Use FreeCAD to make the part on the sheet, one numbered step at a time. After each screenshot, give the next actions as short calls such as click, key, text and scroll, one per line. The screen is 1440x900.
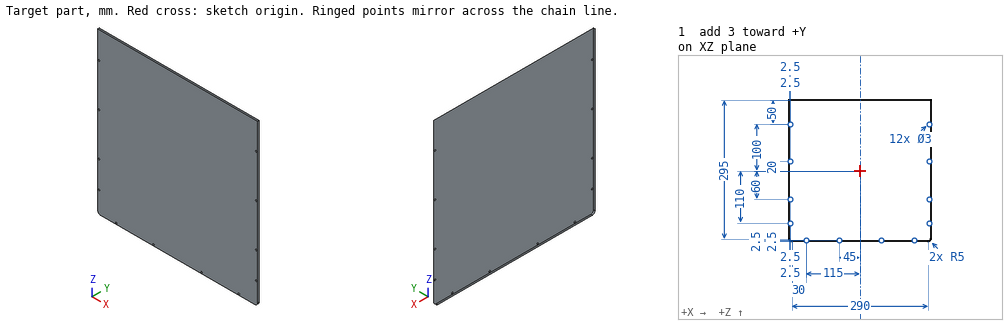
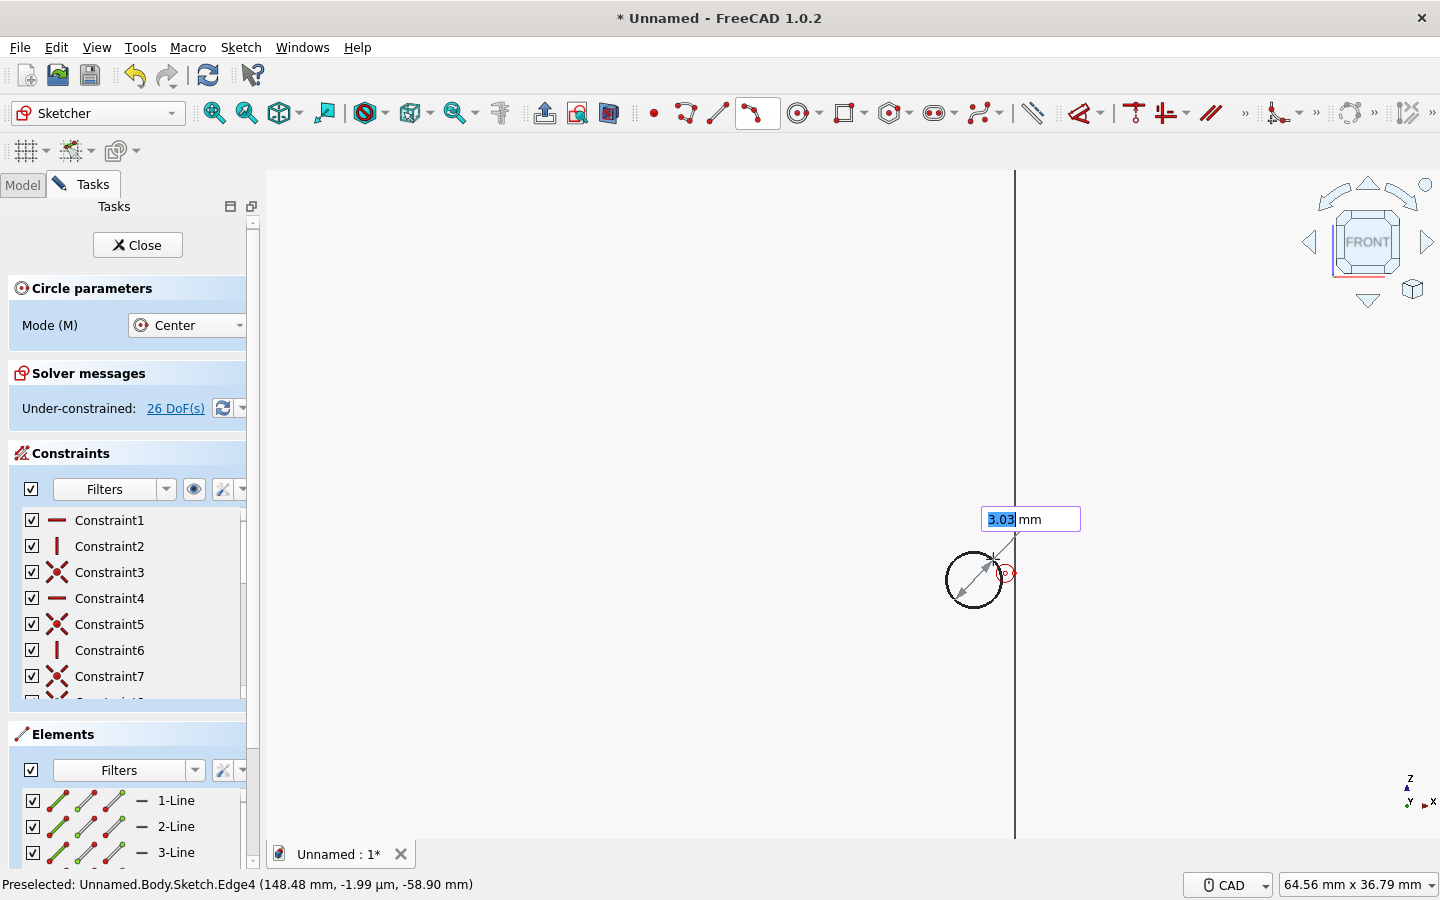
text(3)
key(Return)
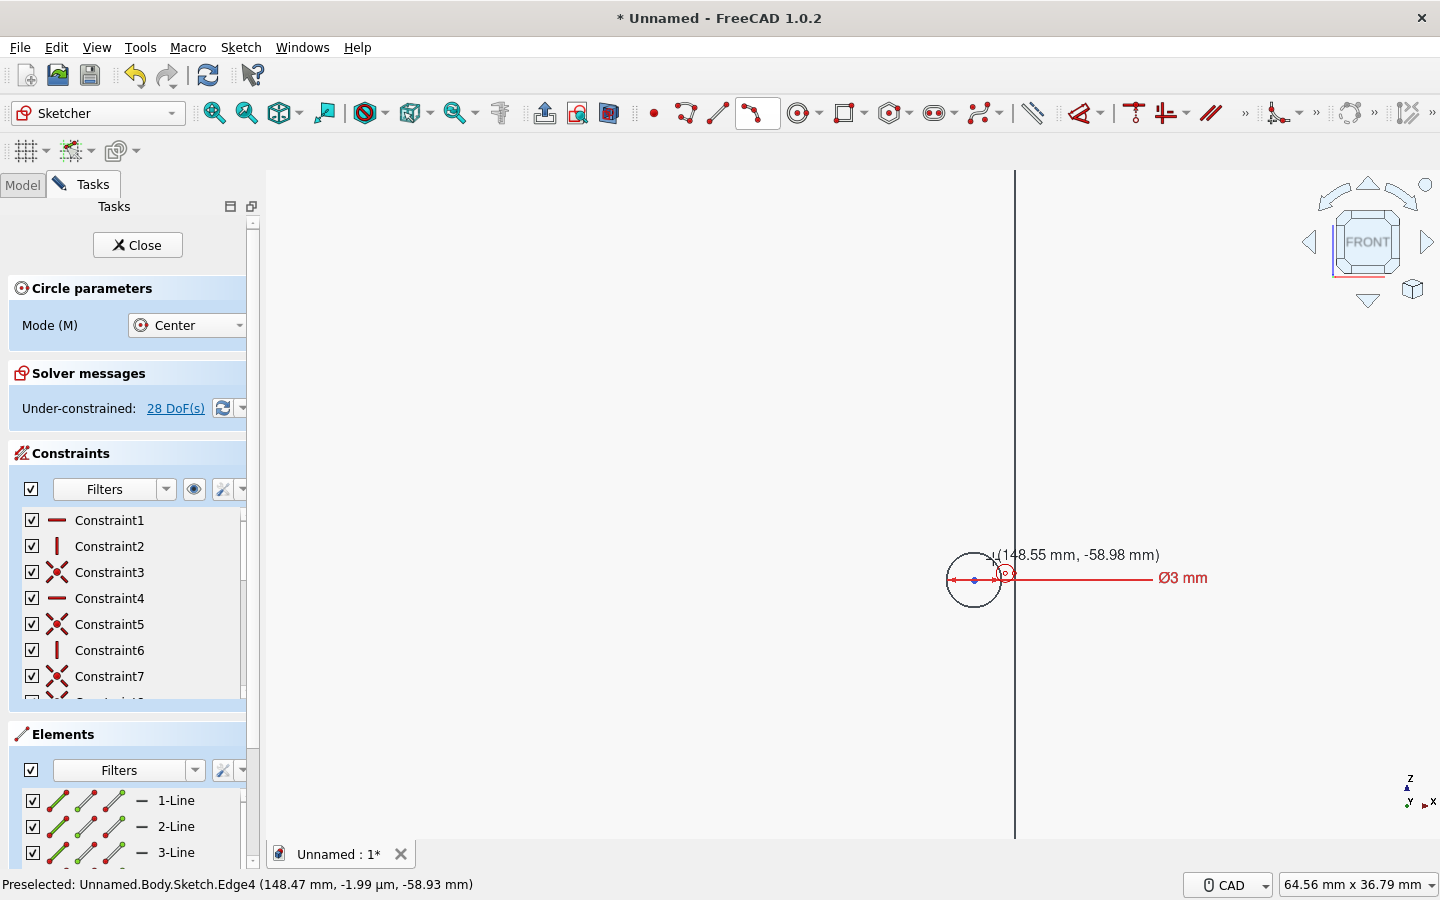
scroll(985, 586, down, 13)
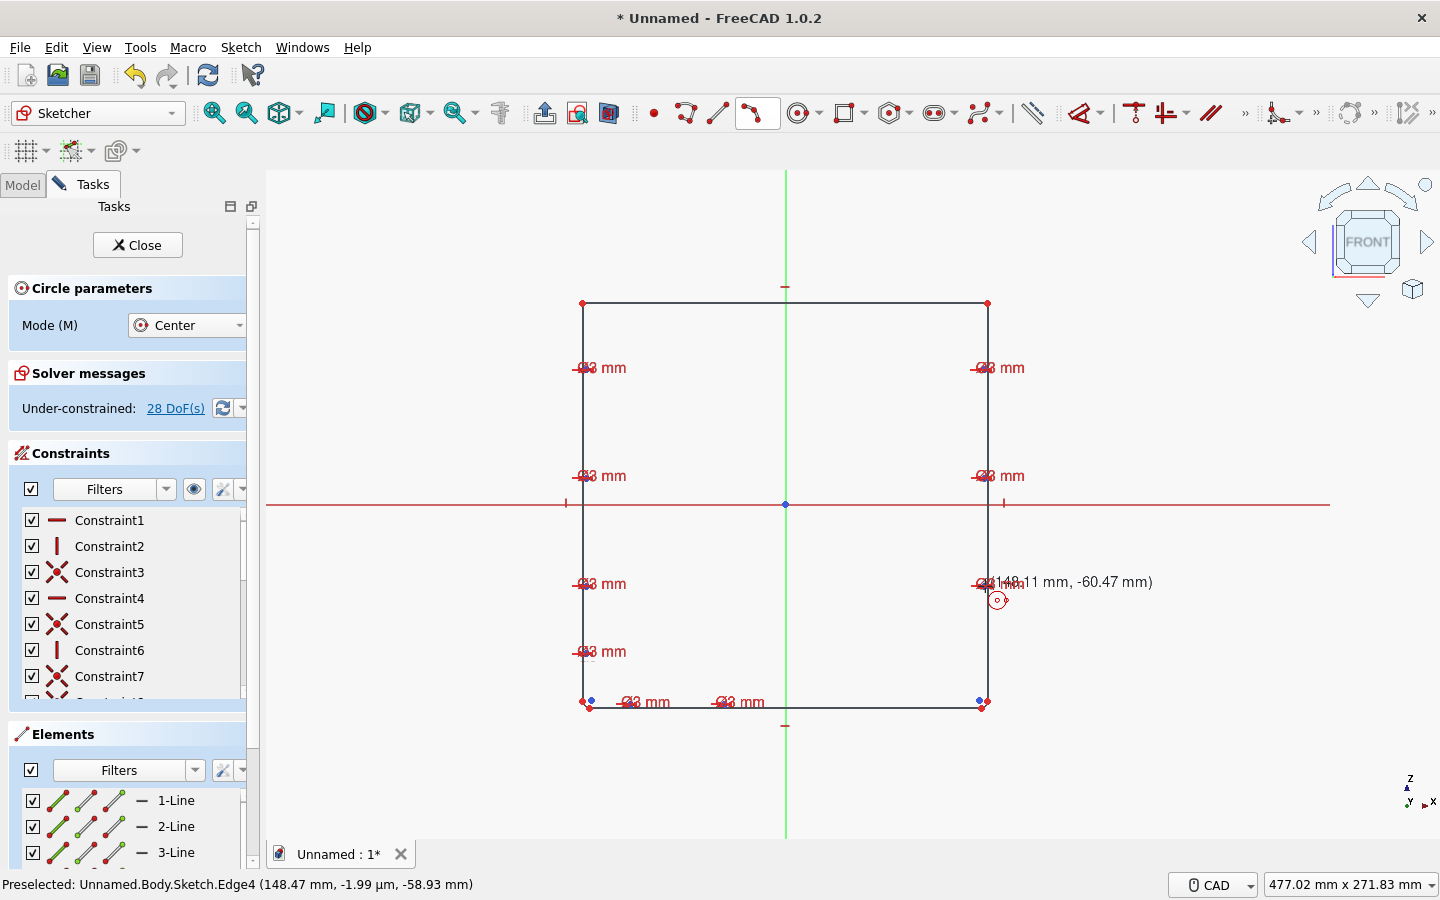
scroll(846, 704, up, 13)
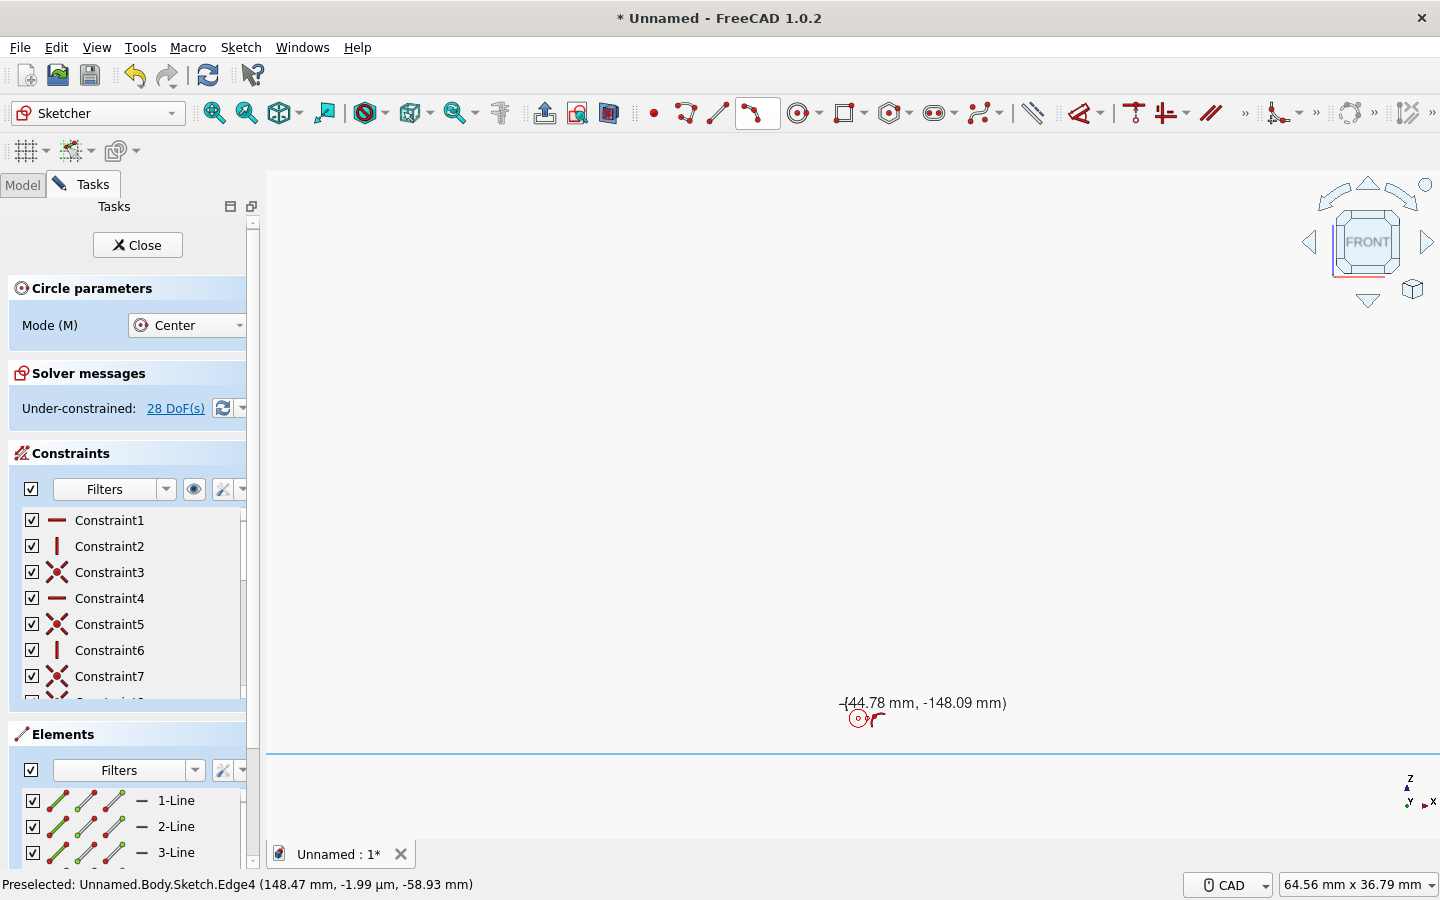
click(844, 697)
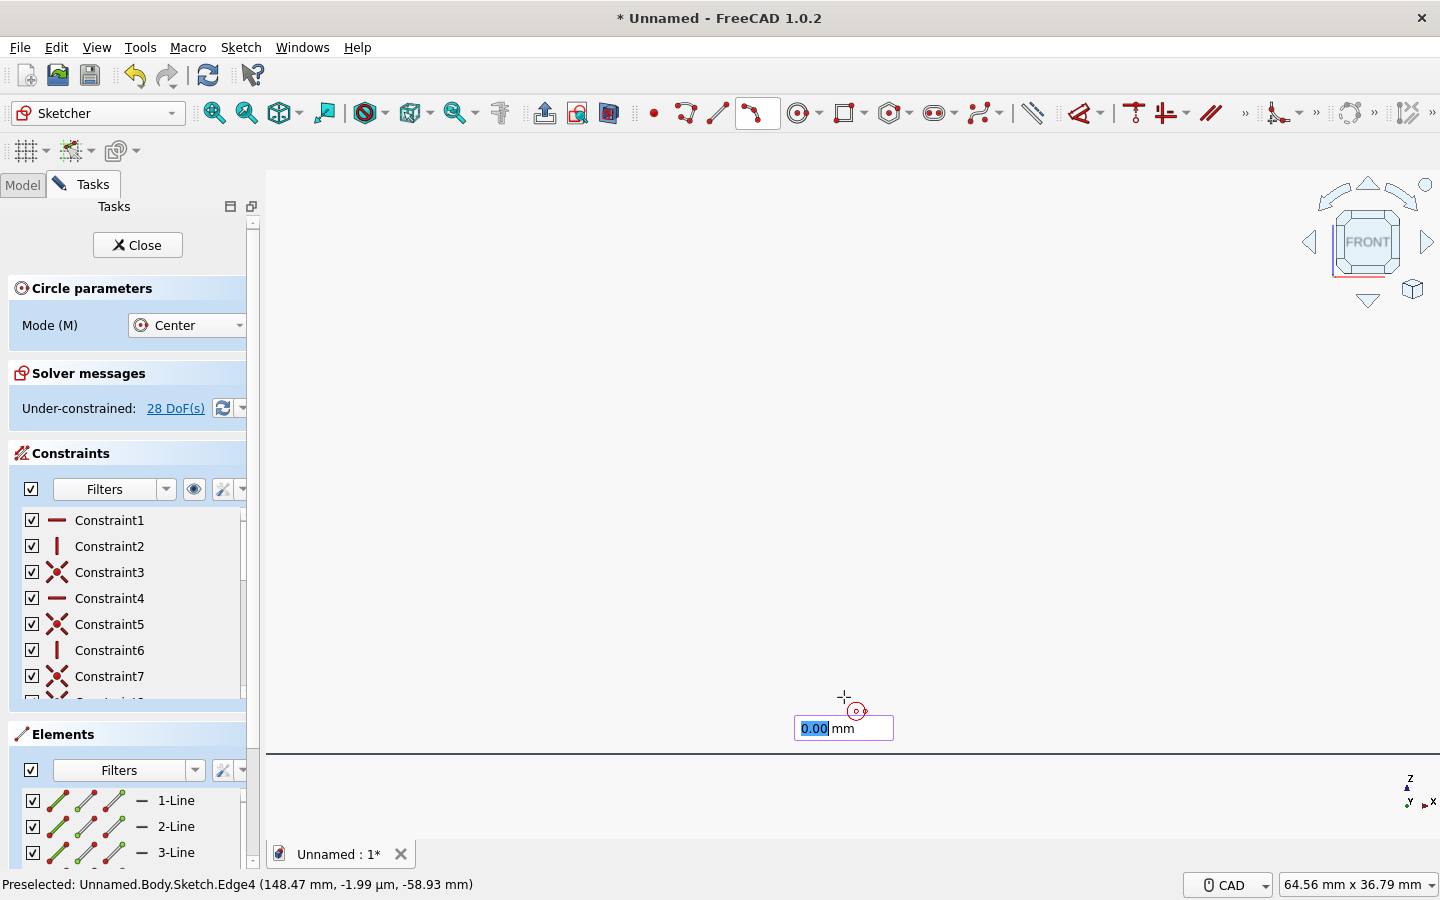
scroll(845, 704, down, 13)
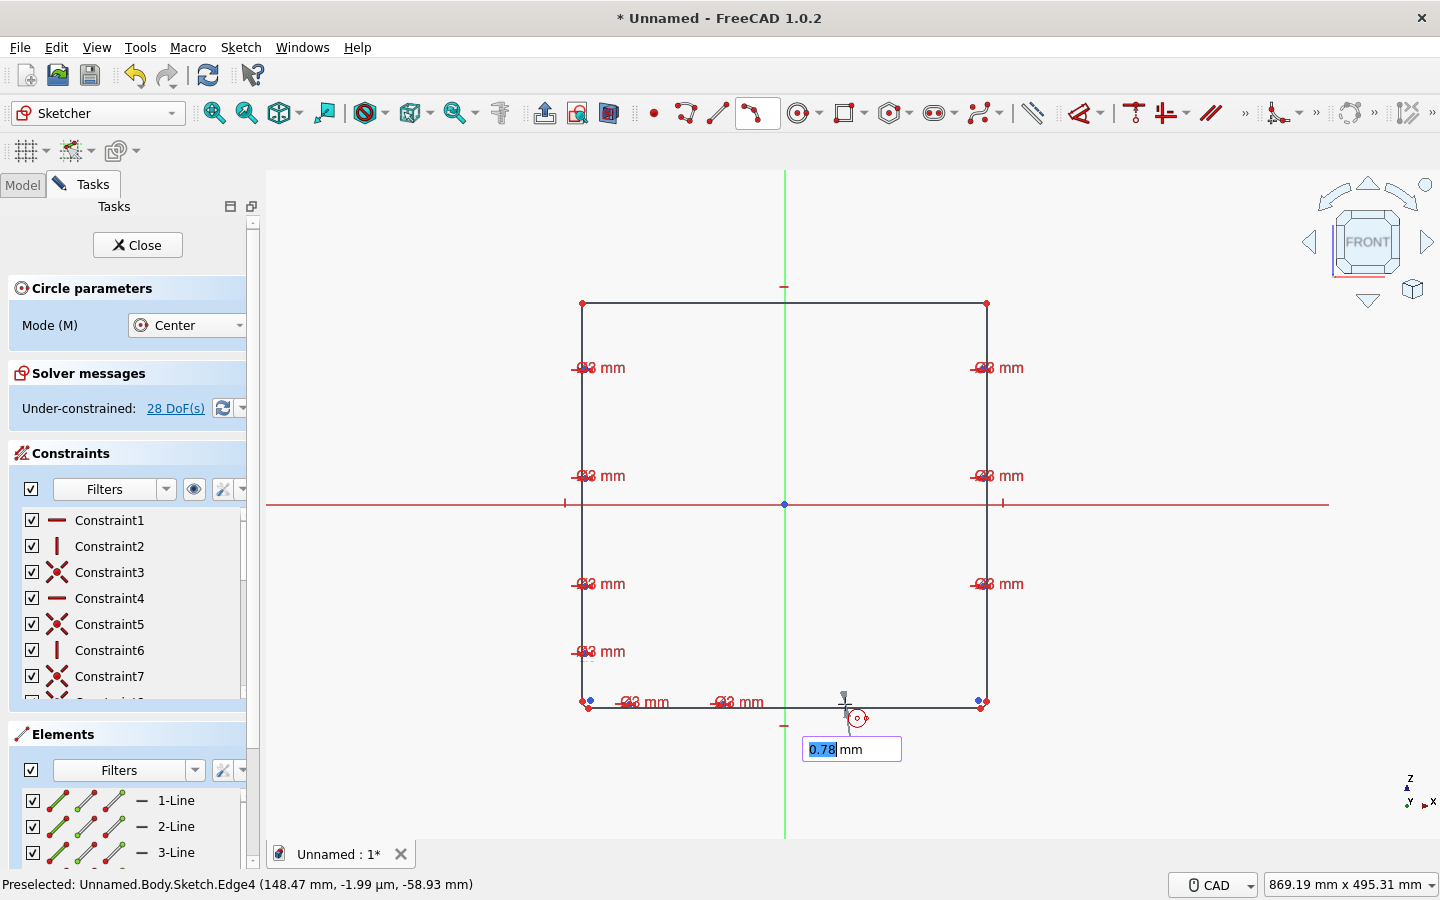
scroll(847, 703, up, 6)
move(845, 700)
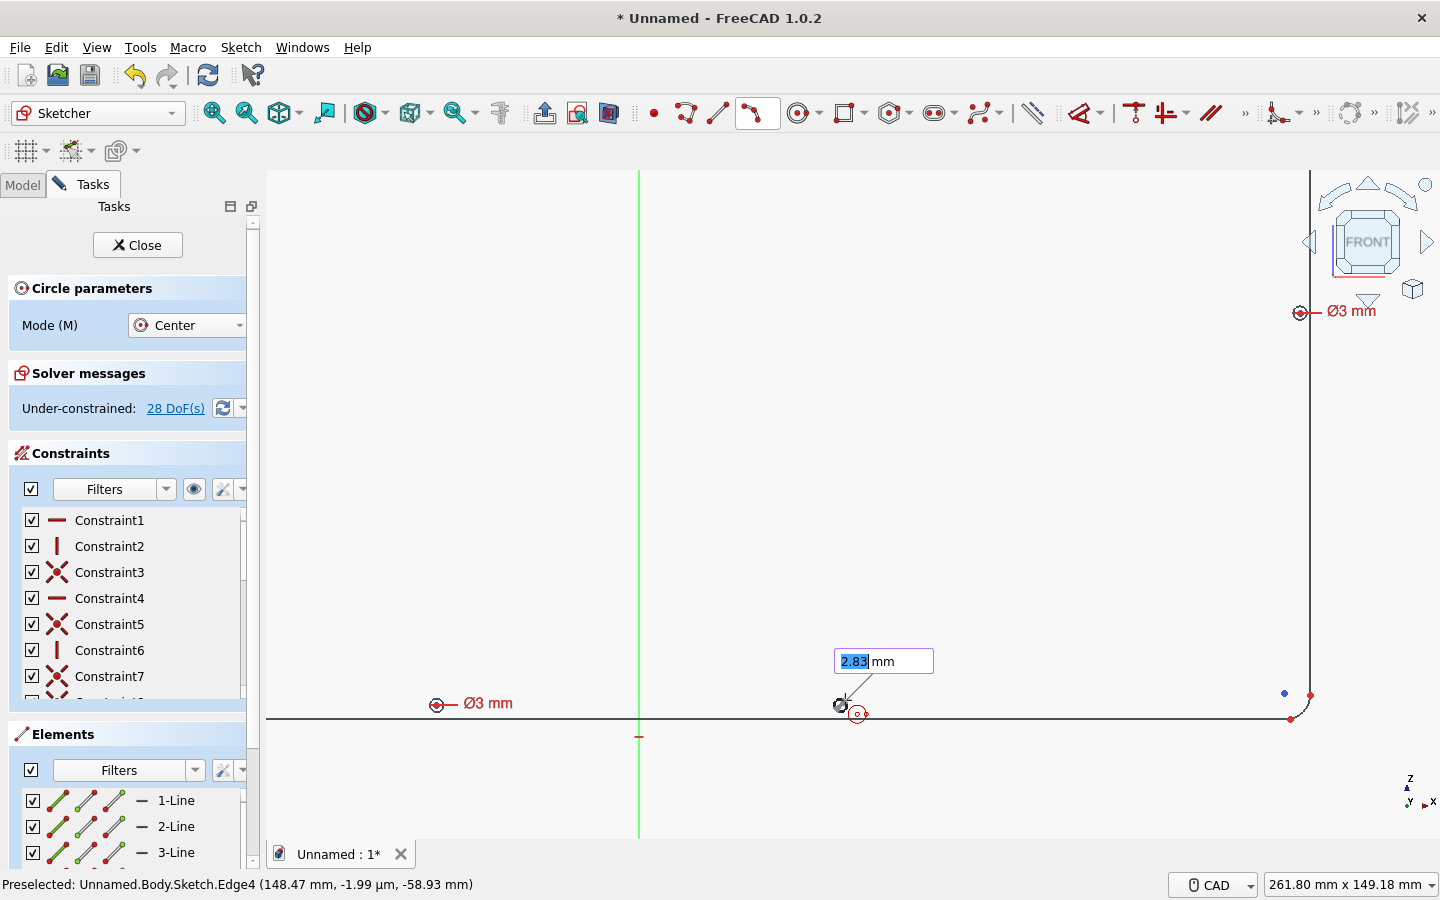
text(3)
key(Return)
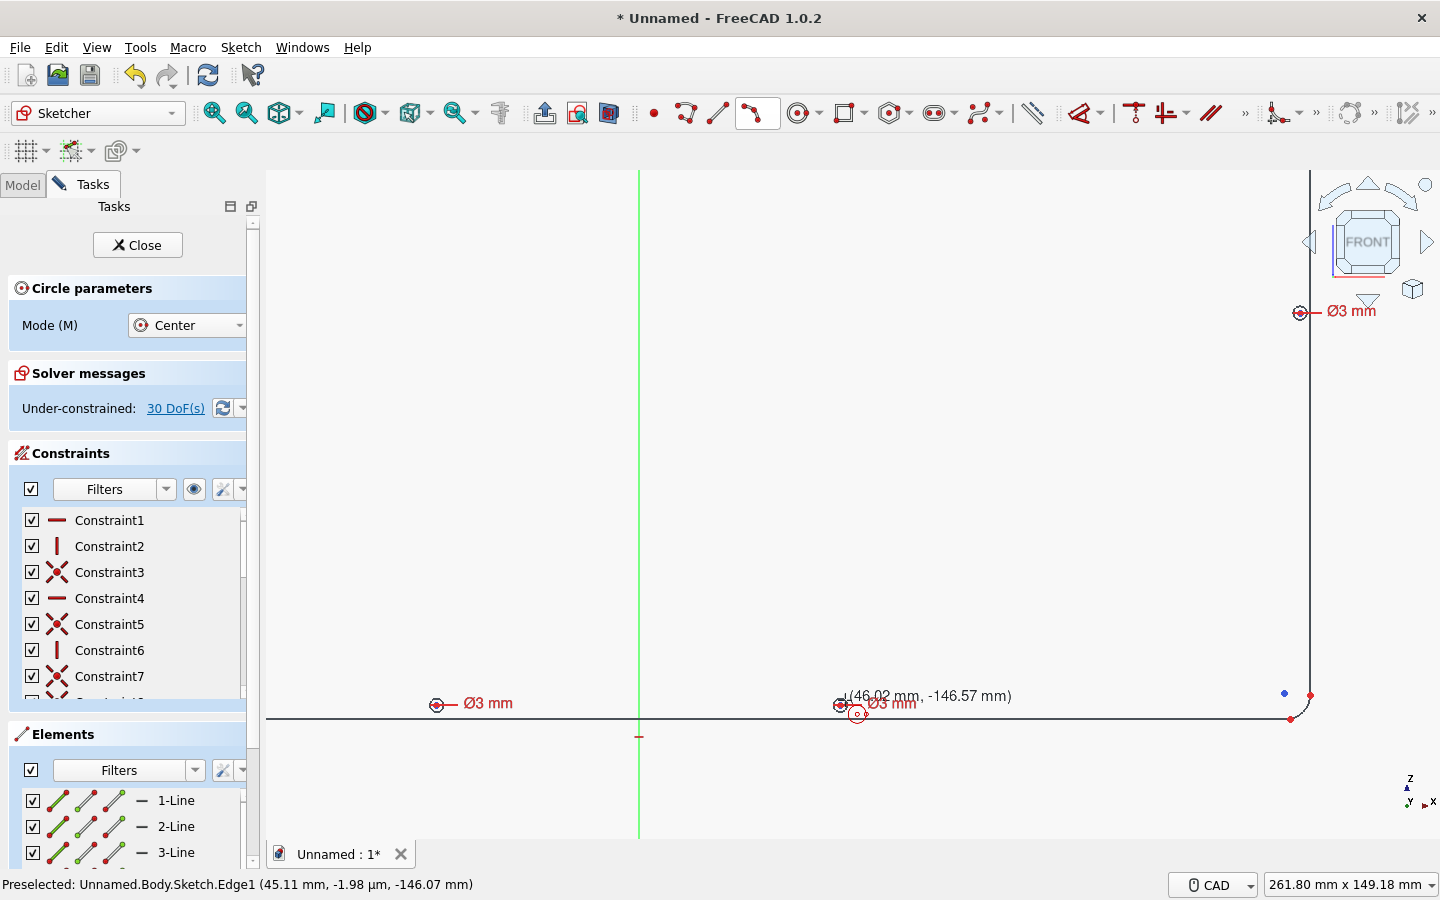
scroll(847, 703, down, 6)